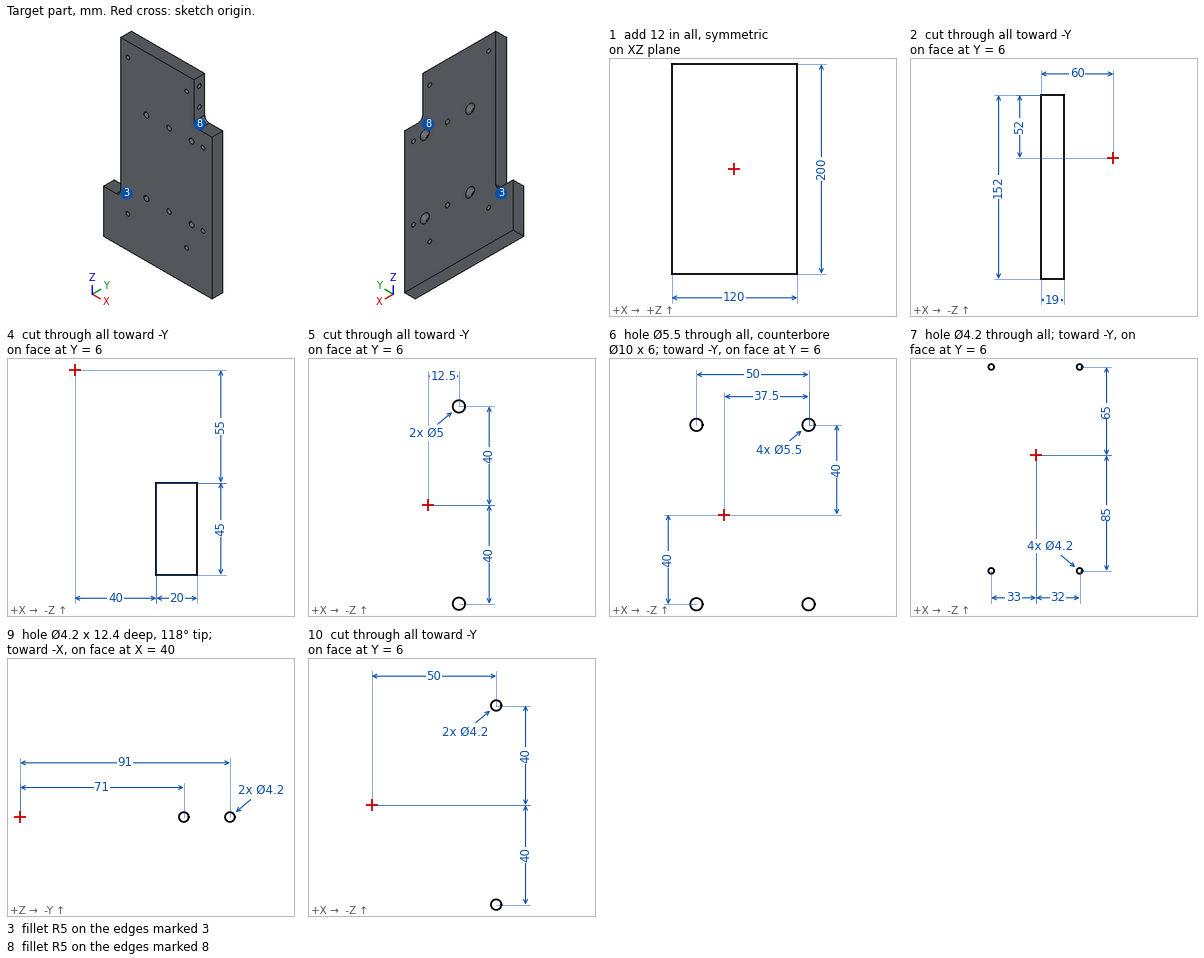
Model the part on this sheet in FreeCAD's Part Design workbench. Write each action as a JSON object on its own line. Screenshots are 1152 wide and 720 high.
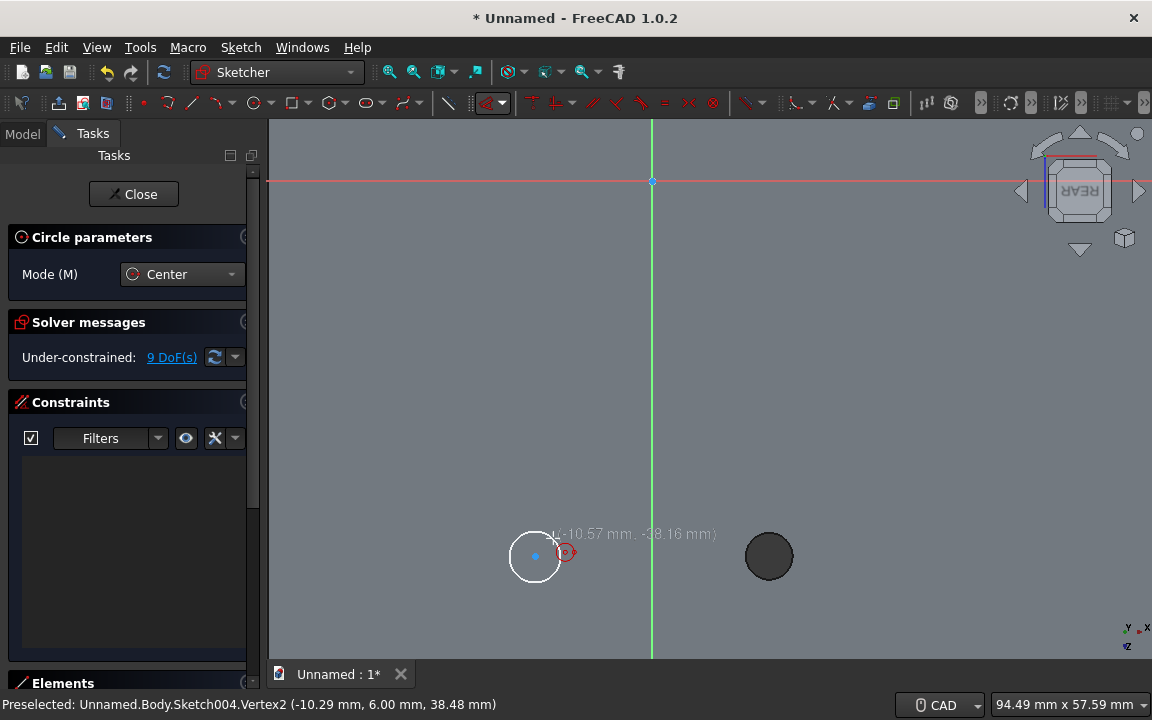
{"action": "scroll", "coordinate": [535, 559], "scroll_direction": "down", "scroll_amount": 4}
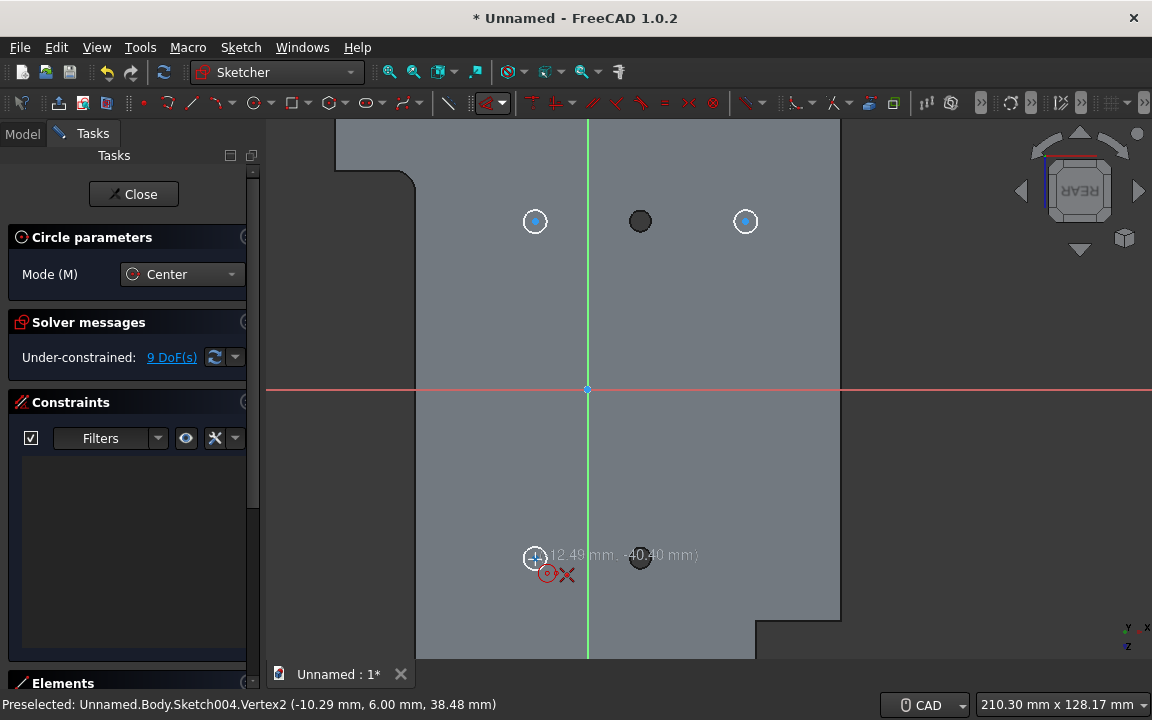
{"action": "scroll", "coordinate": [746, 558], "scroll_direction": "up", "scroll_amount": 4}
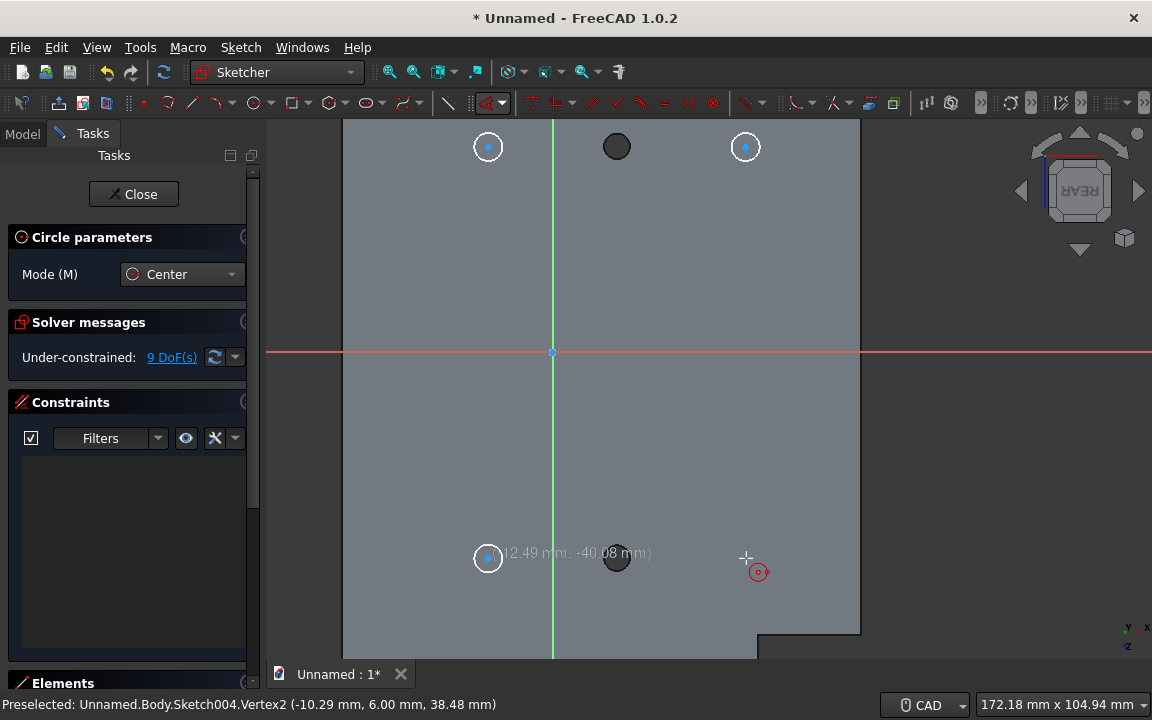
{"action": "left_click", "coordinate": [745, 557]}
{"action": "left_click", "coordinate": [763, 539]}
{"action": "key", "text": "Escape"}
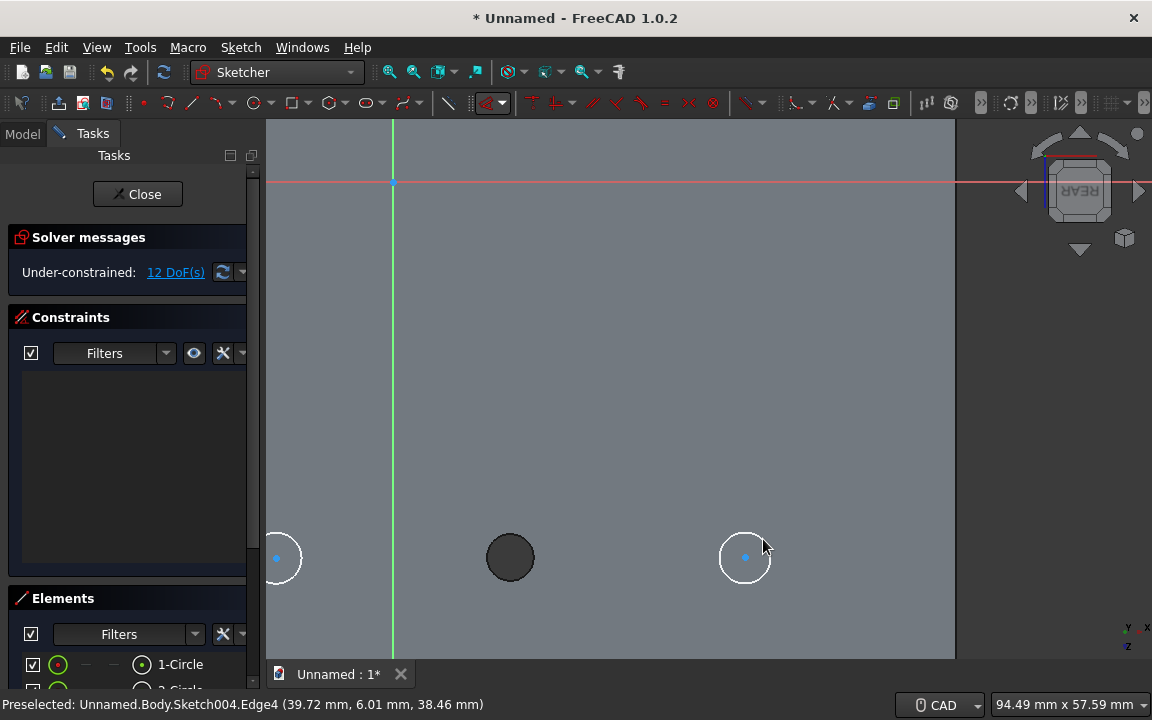
{"action": "scroll", "coordinate": [747, 558], "scroll_direction": "down", "scroll_amount": 4}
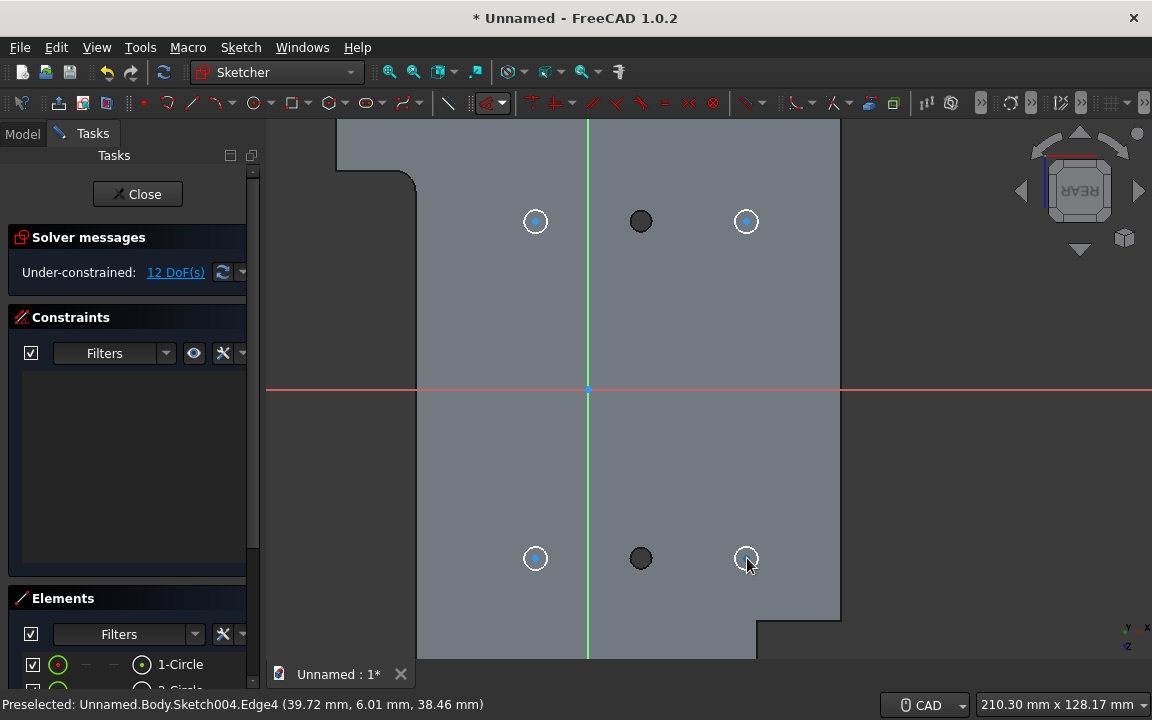
{"action": "left_click", "coordinate": [754, 214]}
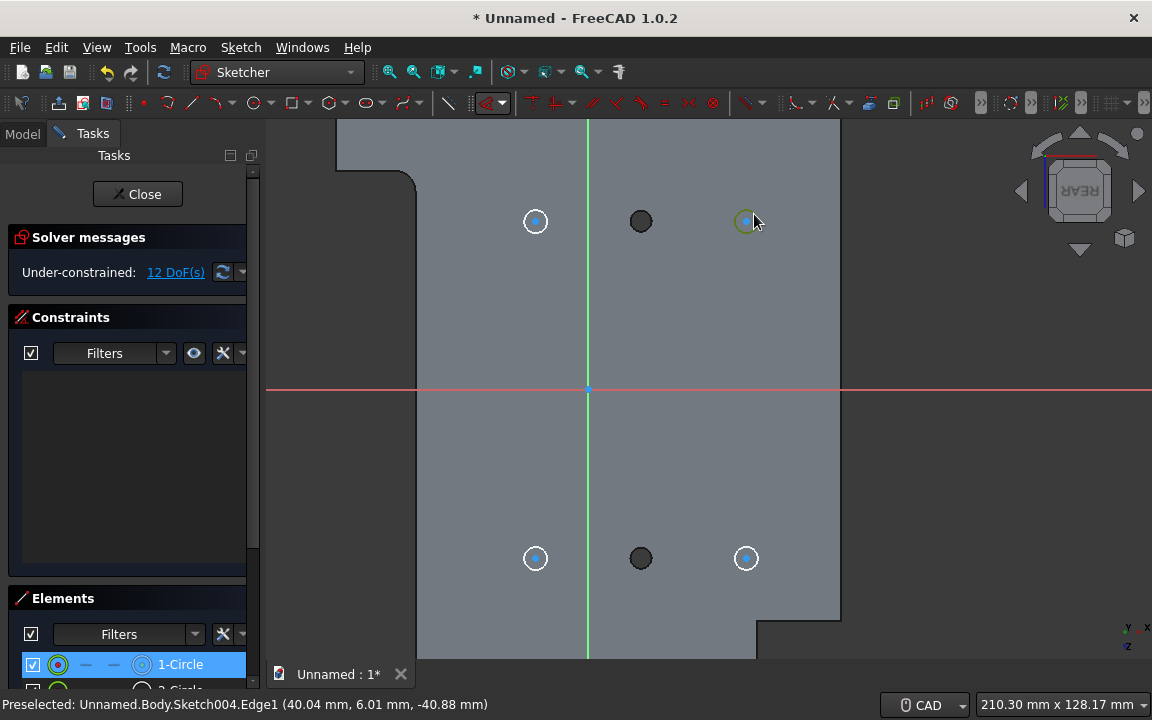
{"action": "left_click", "coordinate": [544, 214]}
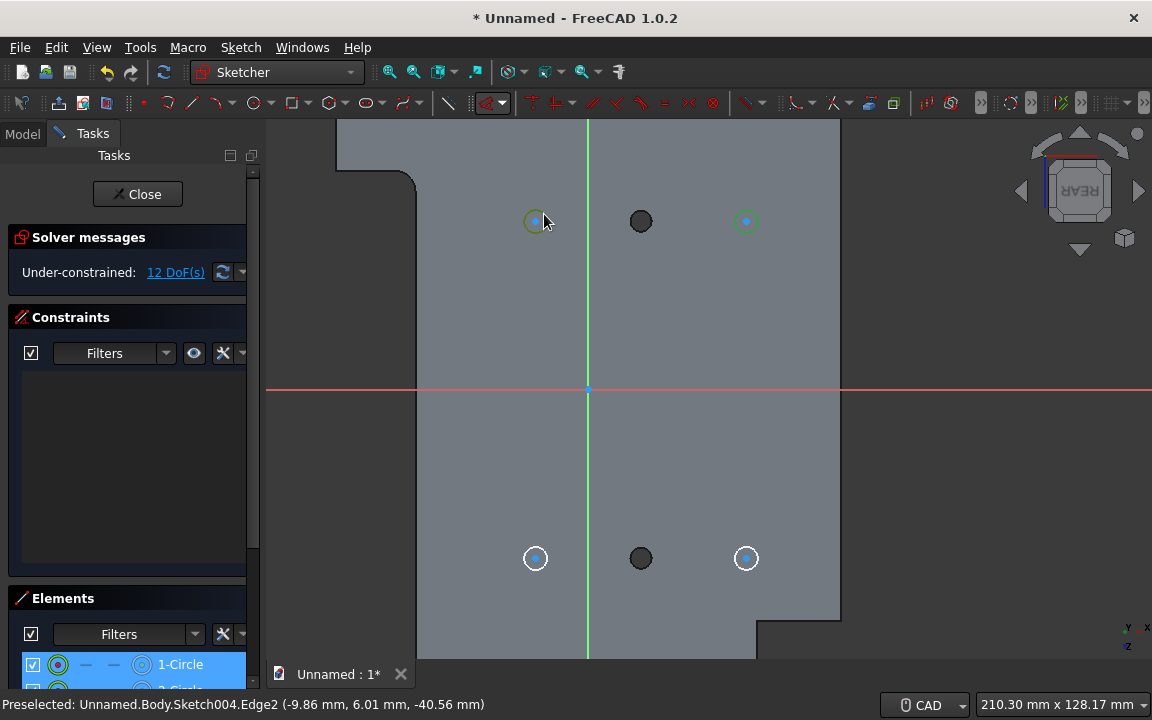
{"action": "left_click", "coordinate": [544, 550]}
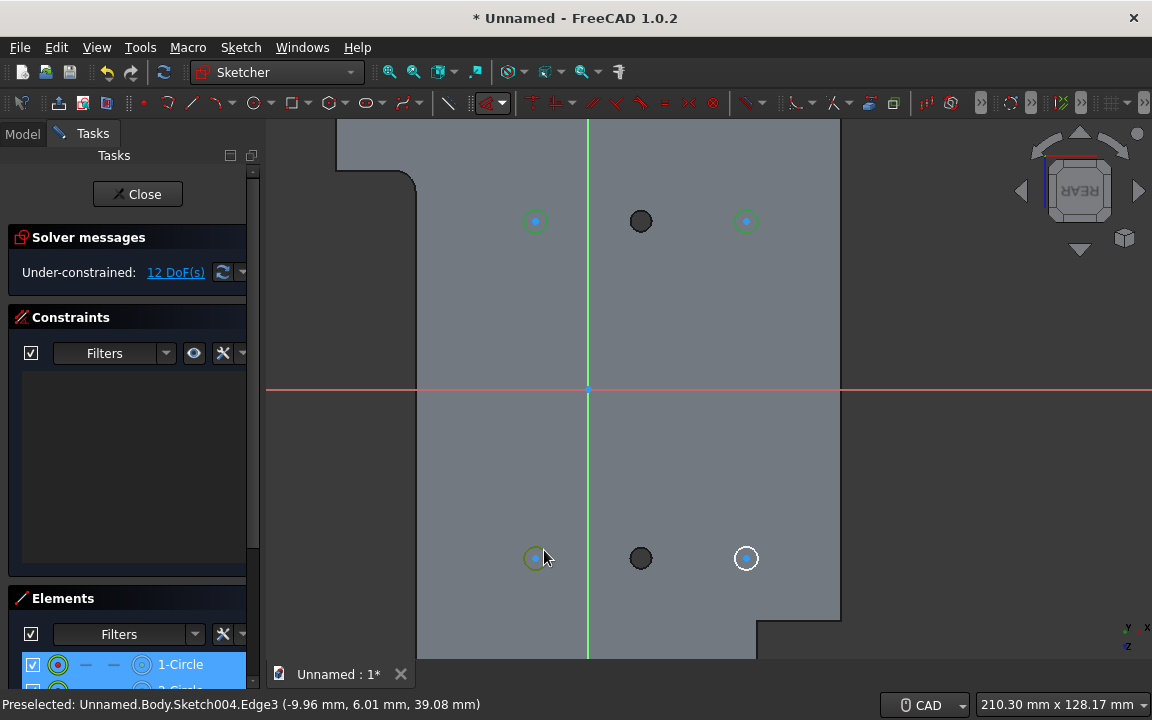
{"action": "left_click", "coordinate": [754, 550]}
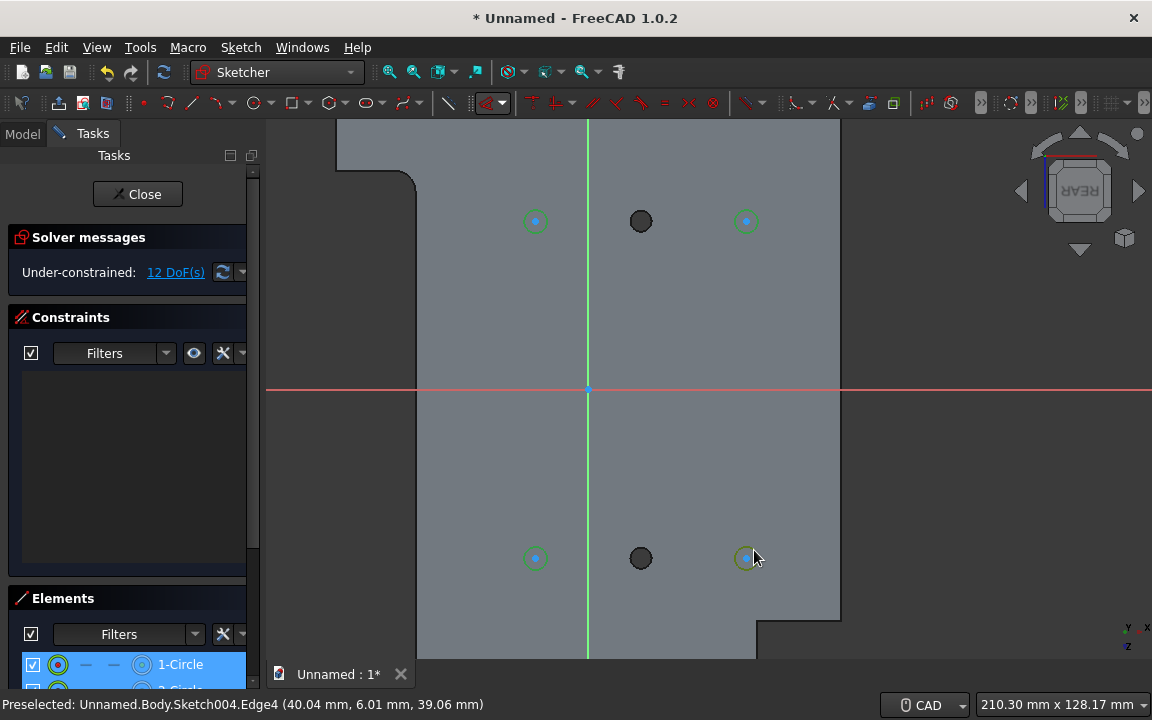
{"action": "left_click", "coordinate": [666, 104]}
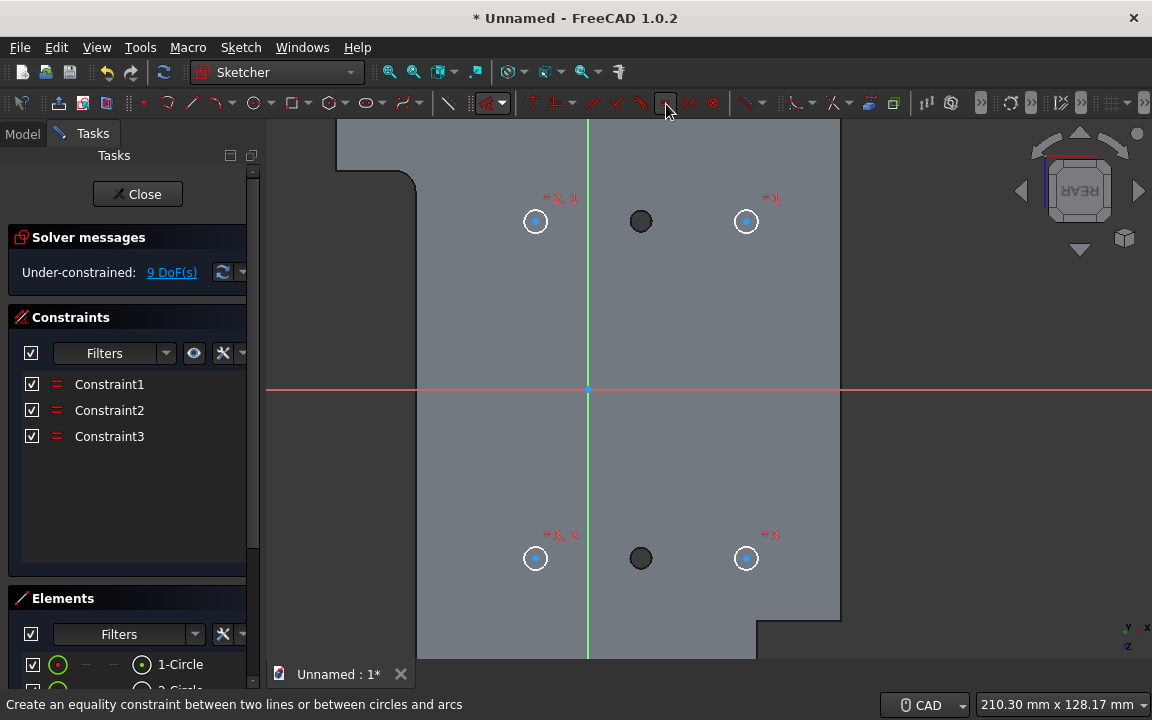
{"action": "left_click", "coordinate": [746, 222]}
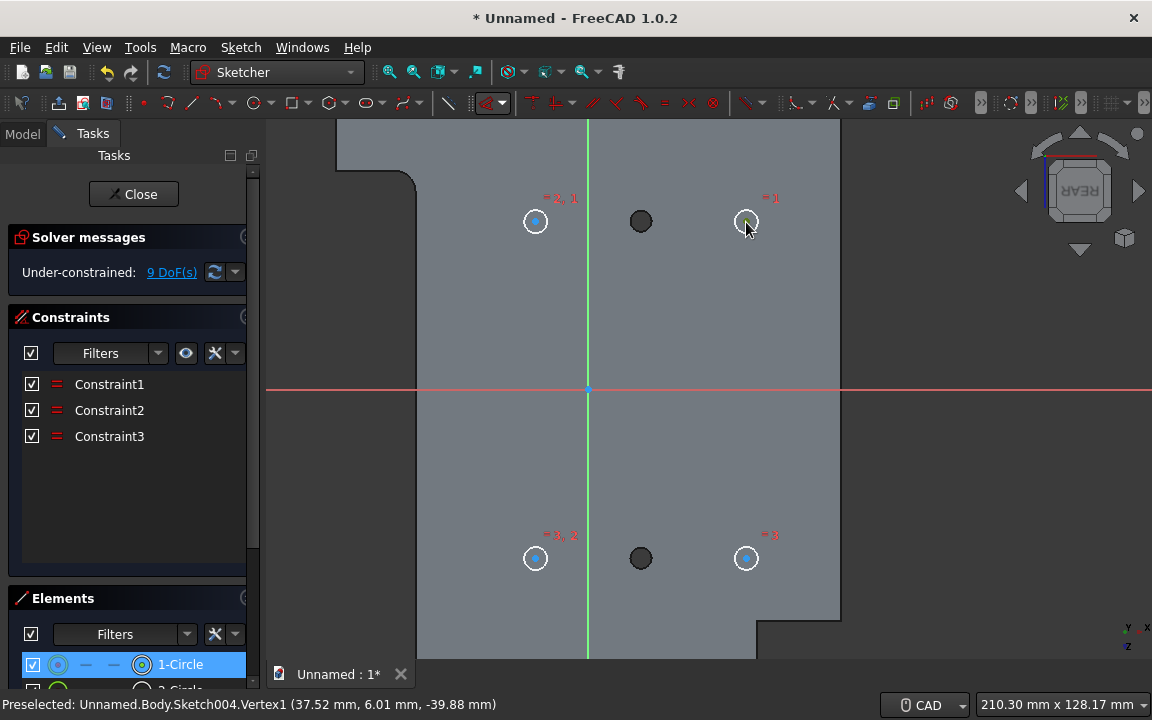
{"action": "left_click", "coordinate": [536, 222]}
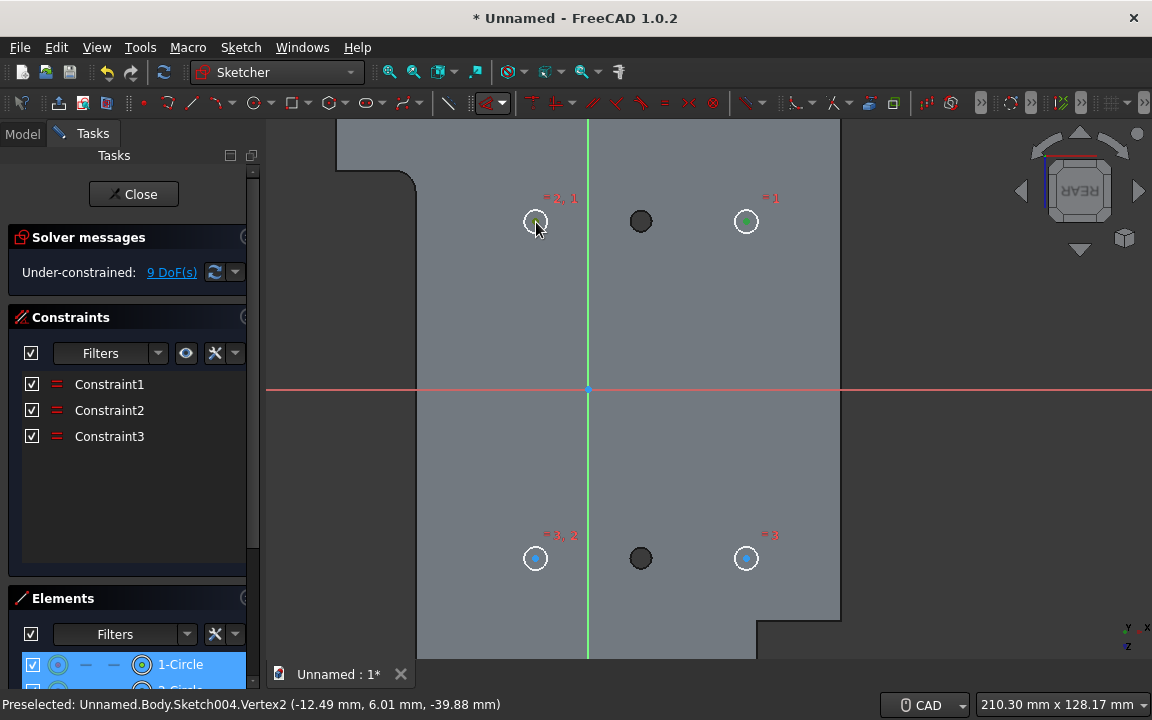
{"action": "key", "text": "h"}